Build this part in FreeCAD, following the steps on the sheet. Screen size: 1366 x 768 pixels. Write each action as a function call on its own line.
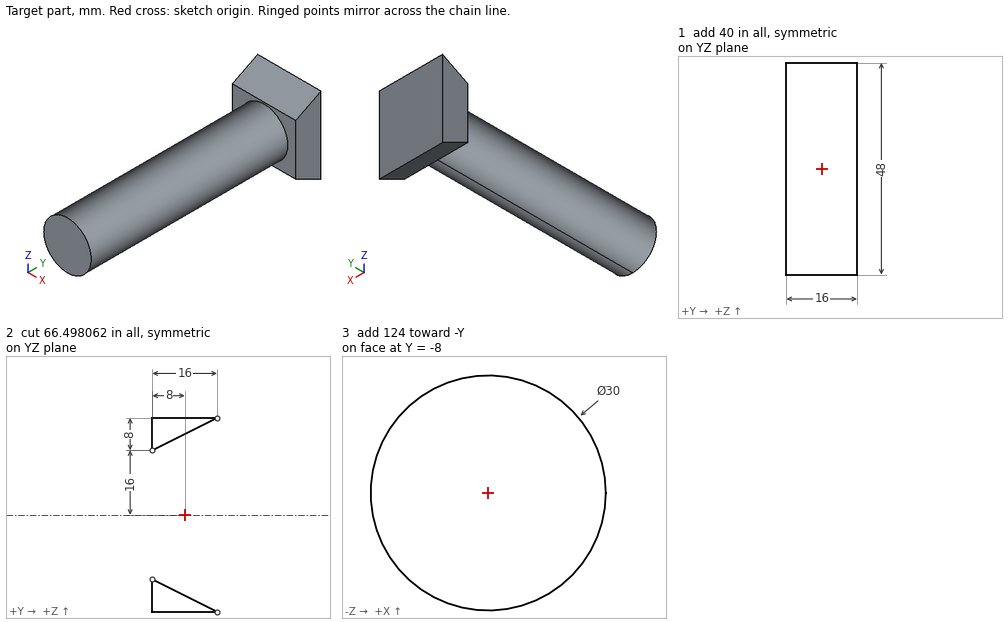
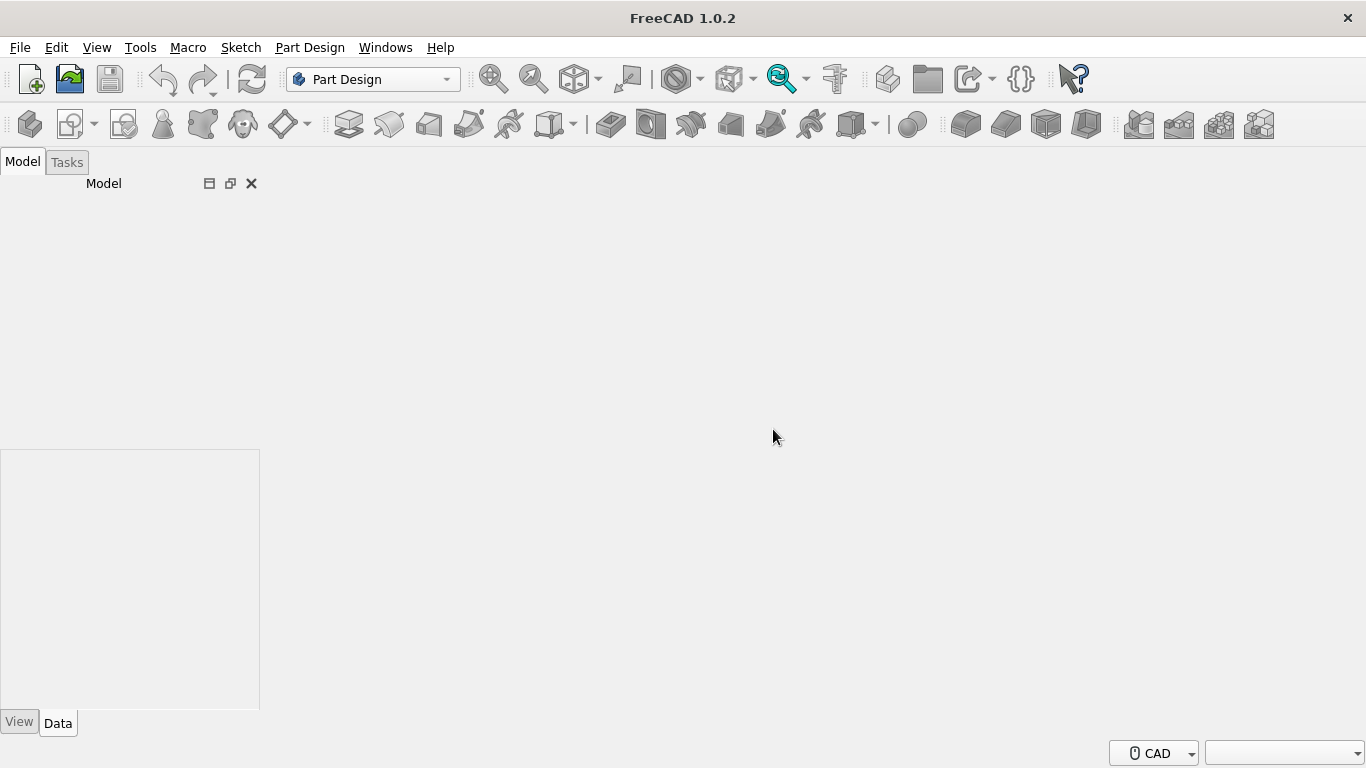
click(30, 80)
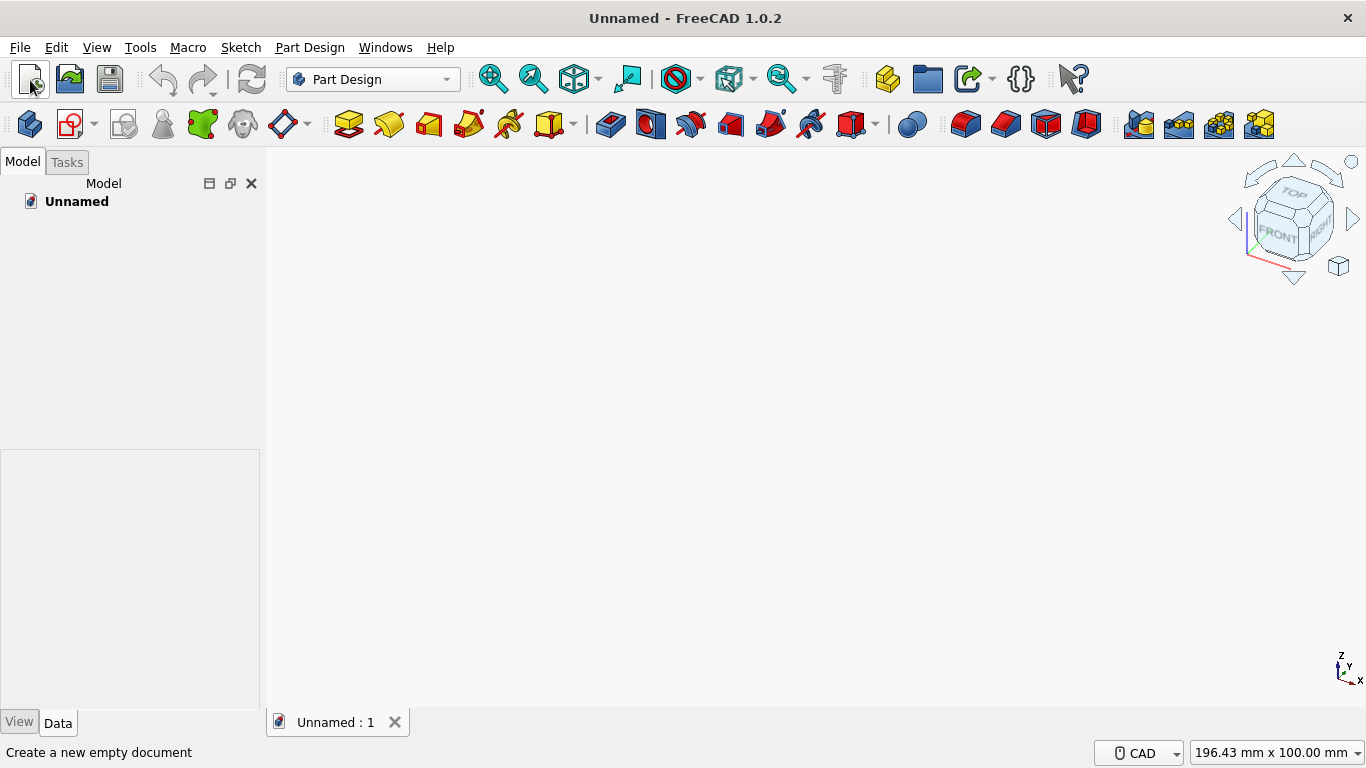
click(70, 124)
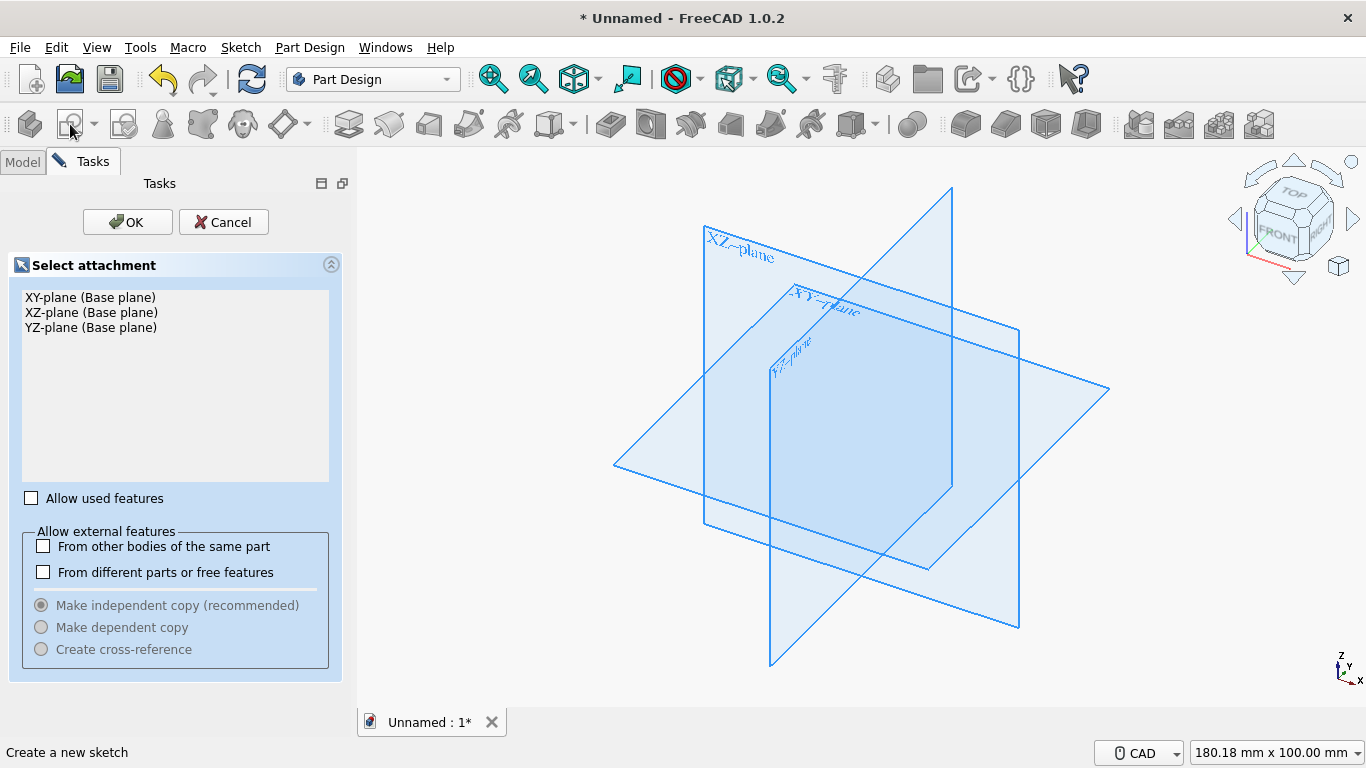
click(82, 328)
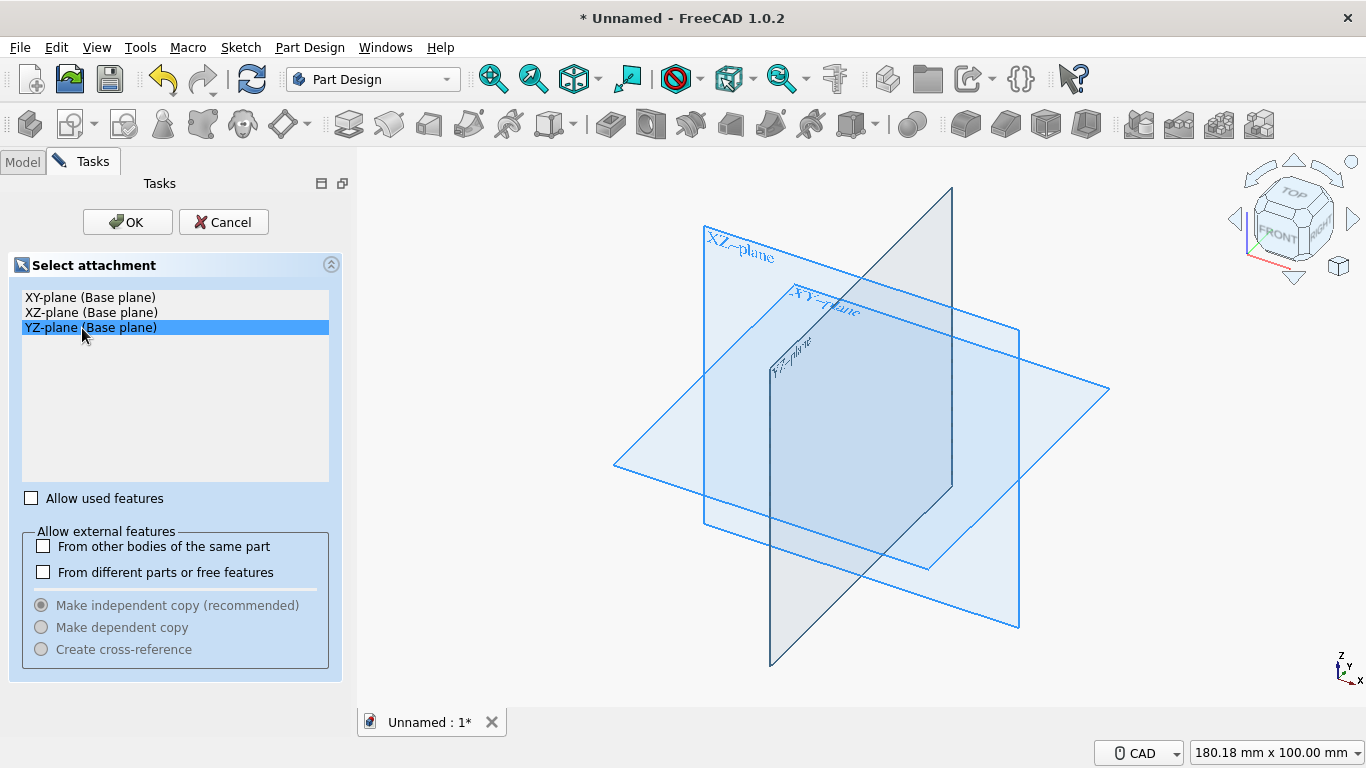
click(128, 222)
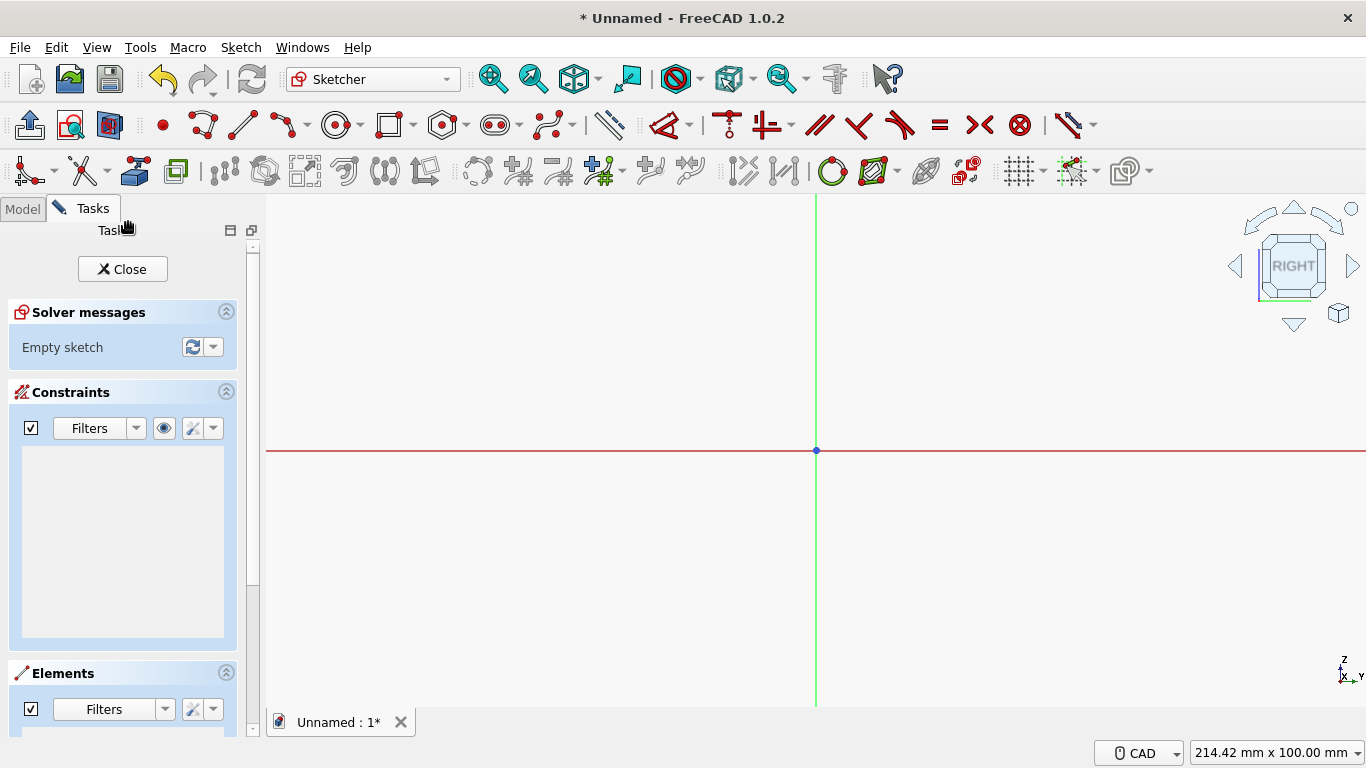
click(416, 126)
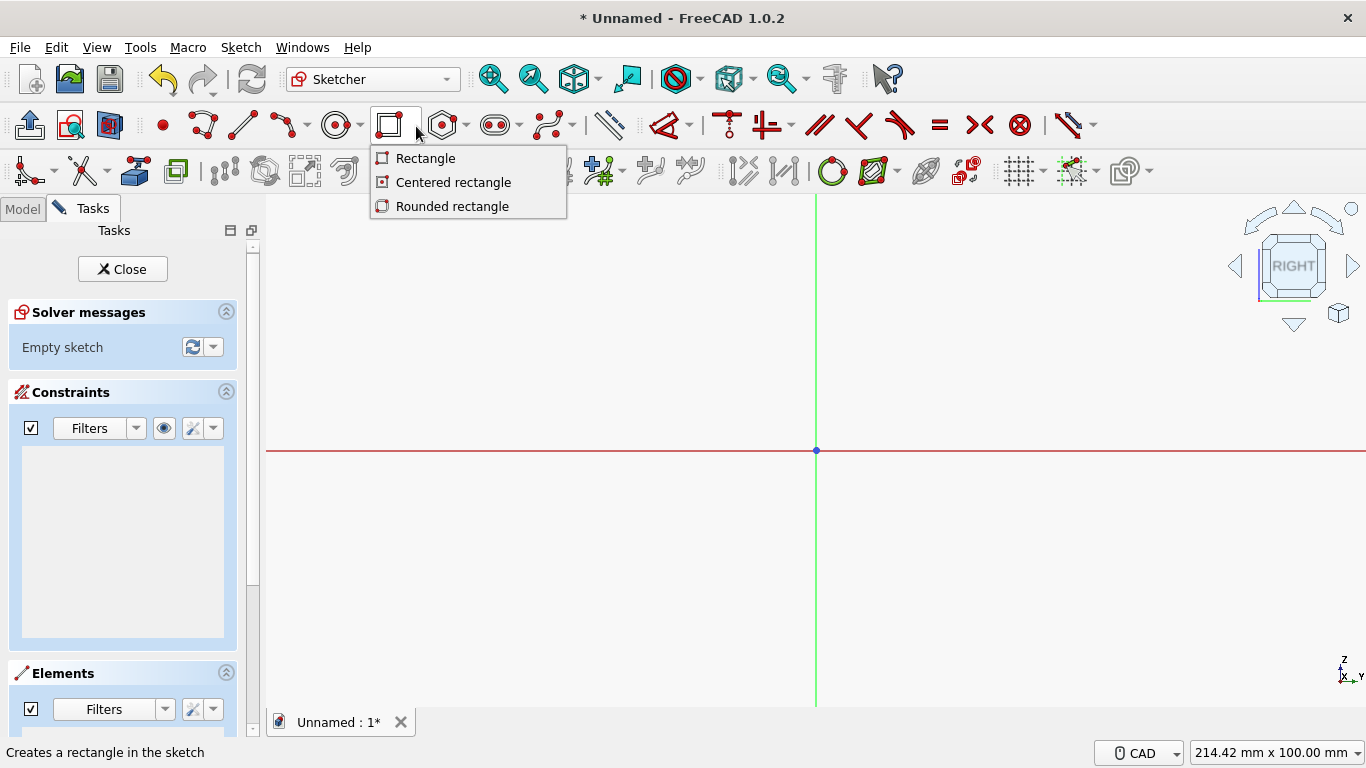
click(468, 182)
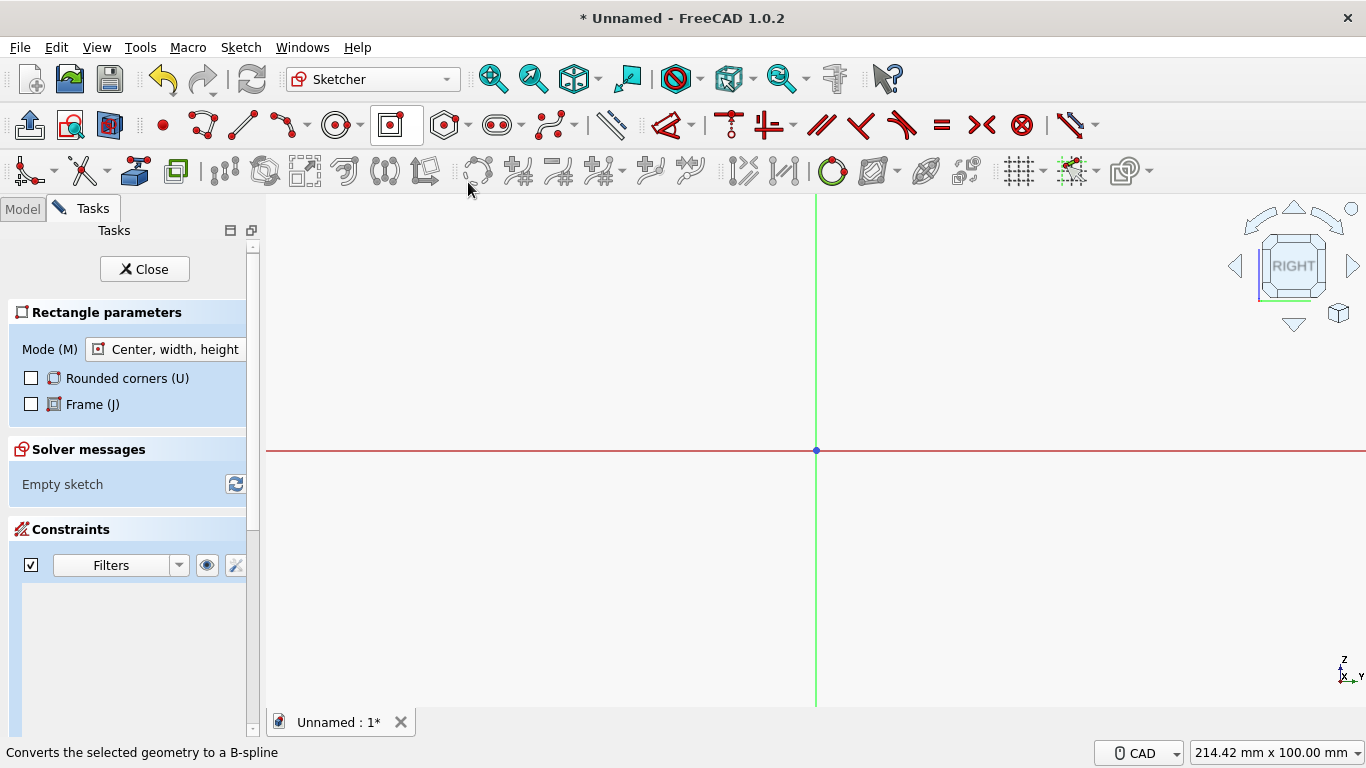
click(816, 450)
move(857, 327)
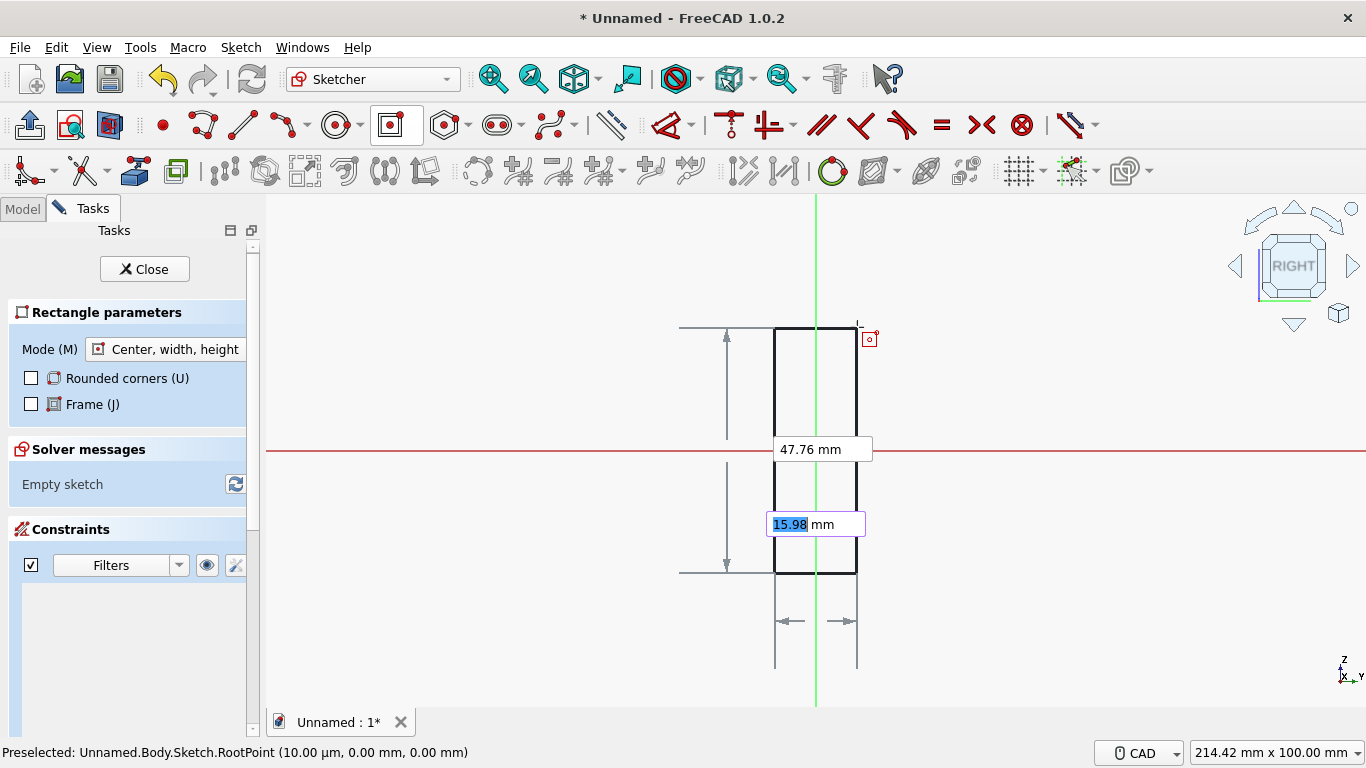
text(16)
key(Tab)
text(48)
key(Return)
key(Escape)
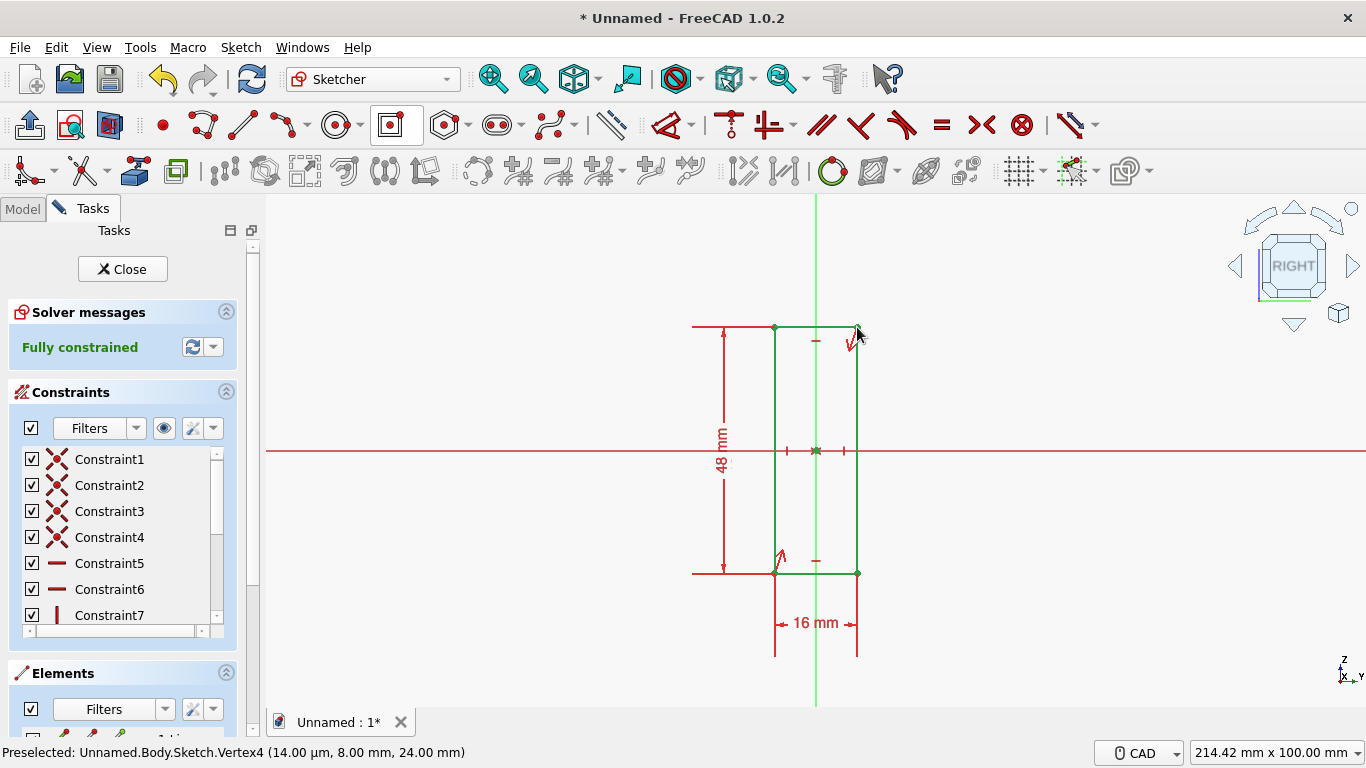
click(123, 269)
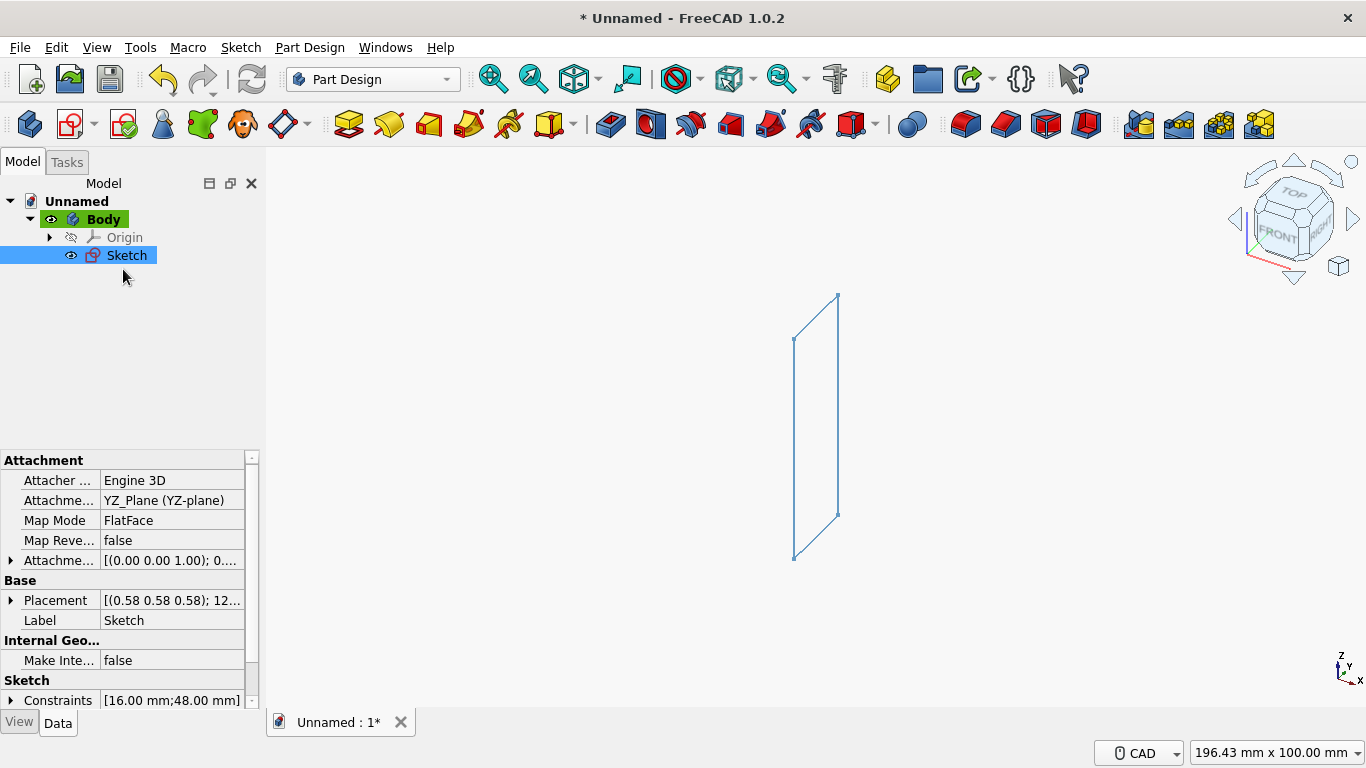
click(350, 124)